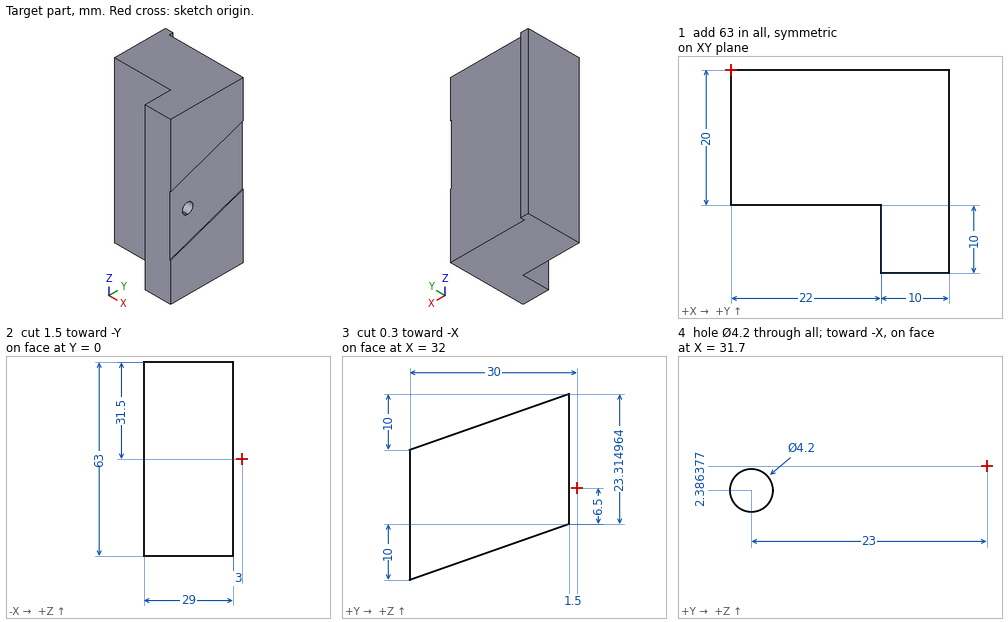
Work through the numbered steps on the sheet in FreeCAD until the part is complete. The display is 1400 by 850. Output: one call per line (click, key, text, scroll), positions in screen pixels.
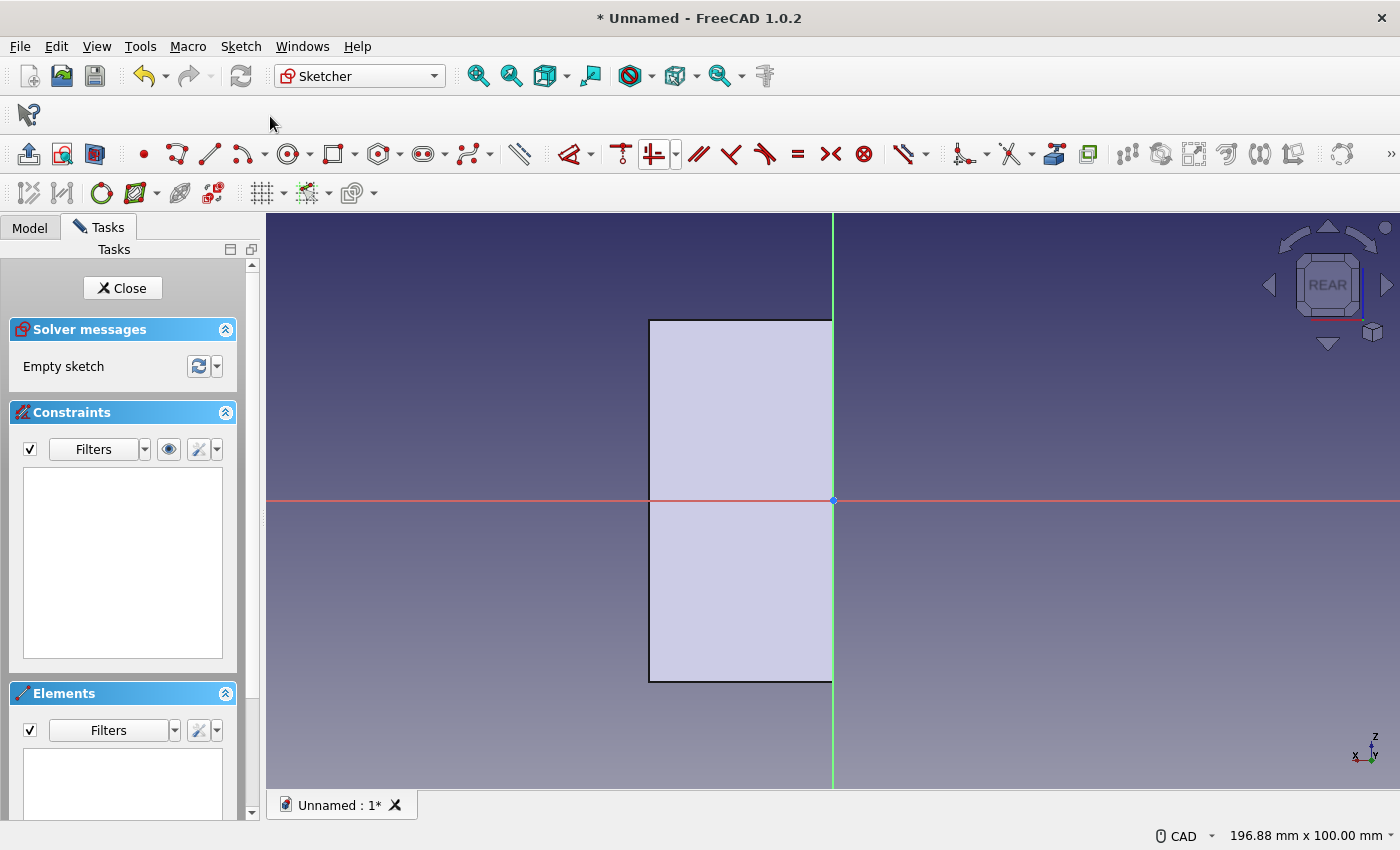
click(332, 154)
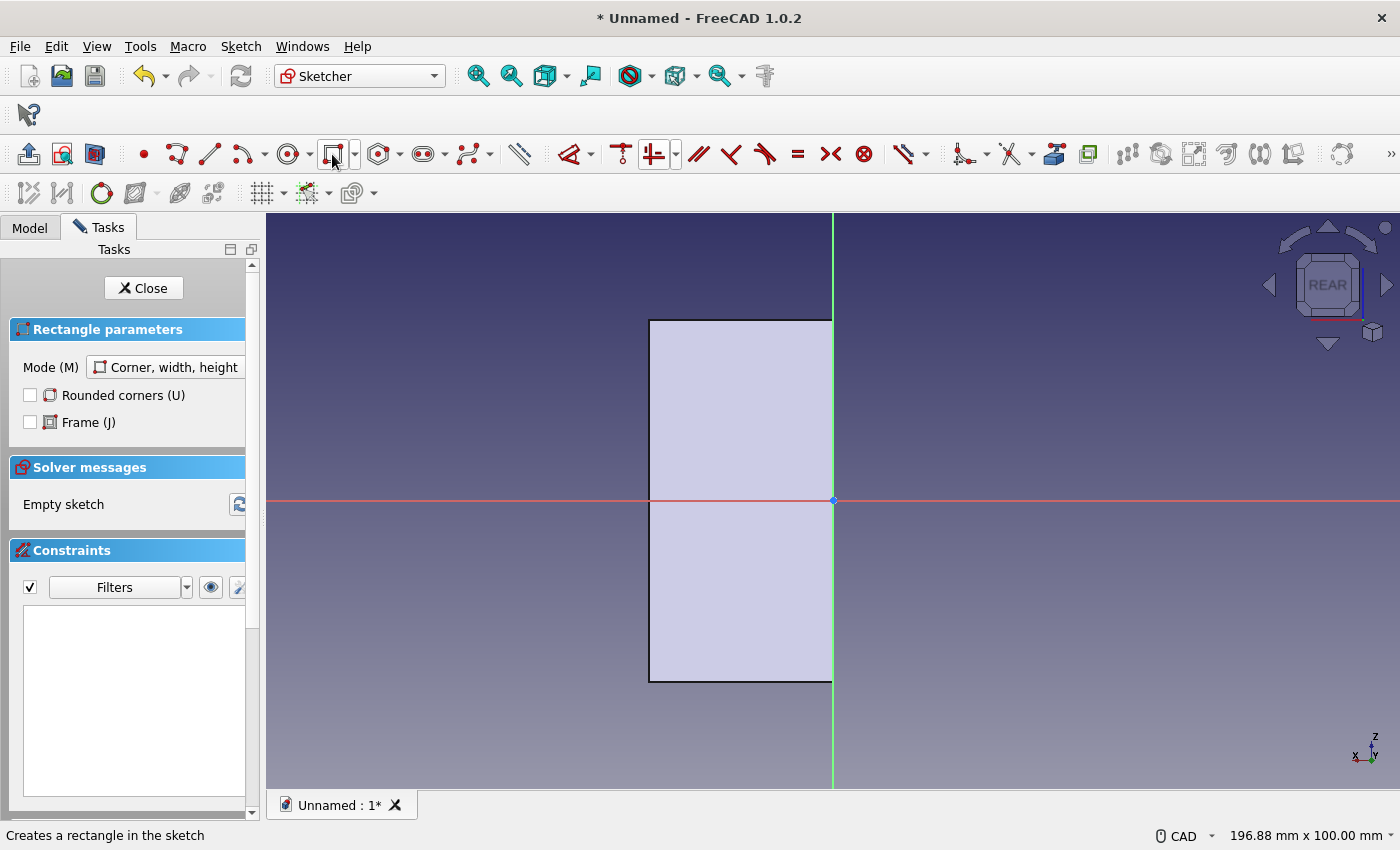
click(649, 320)
click(816, 682)
key(Escape)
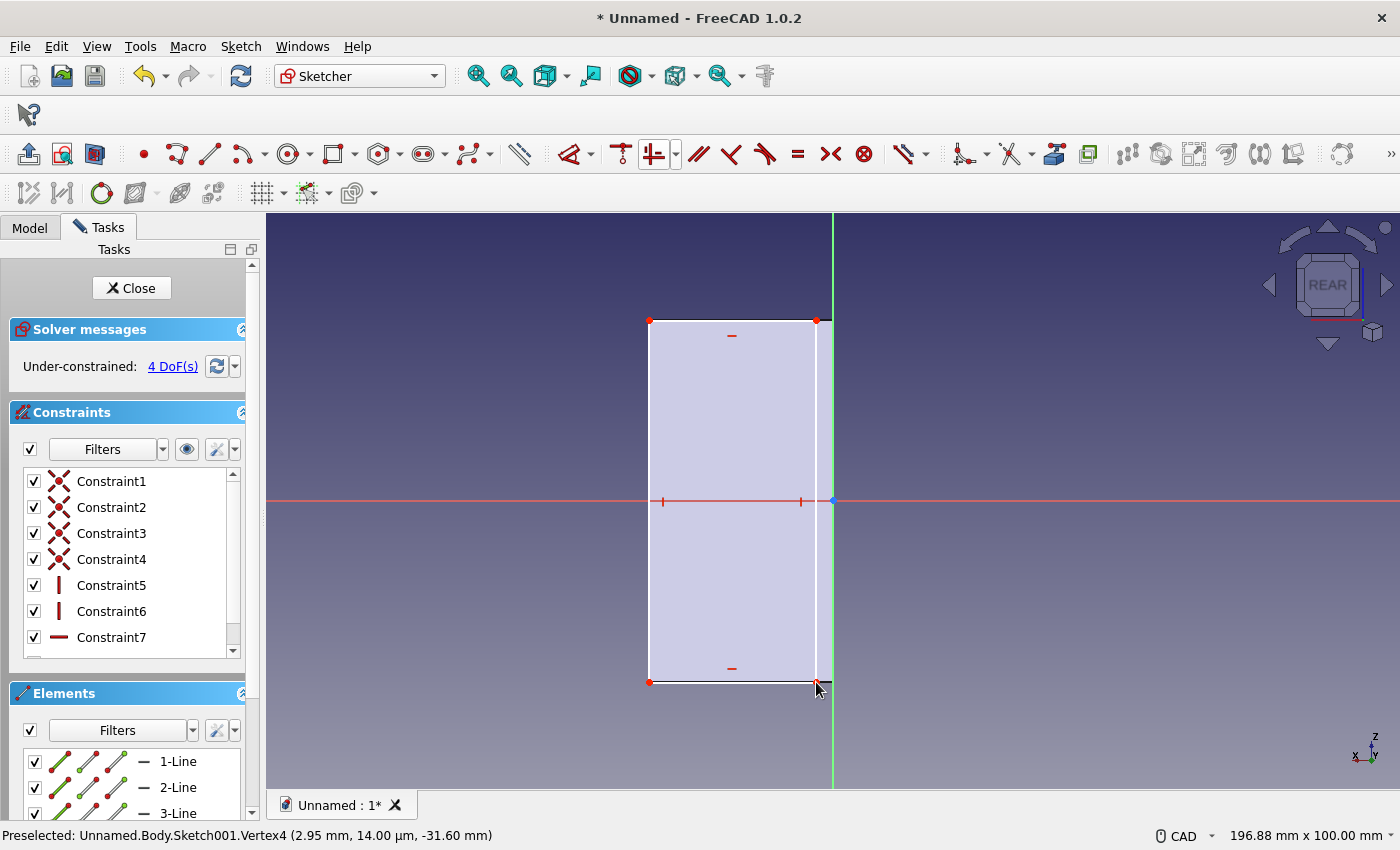
click(568, 154)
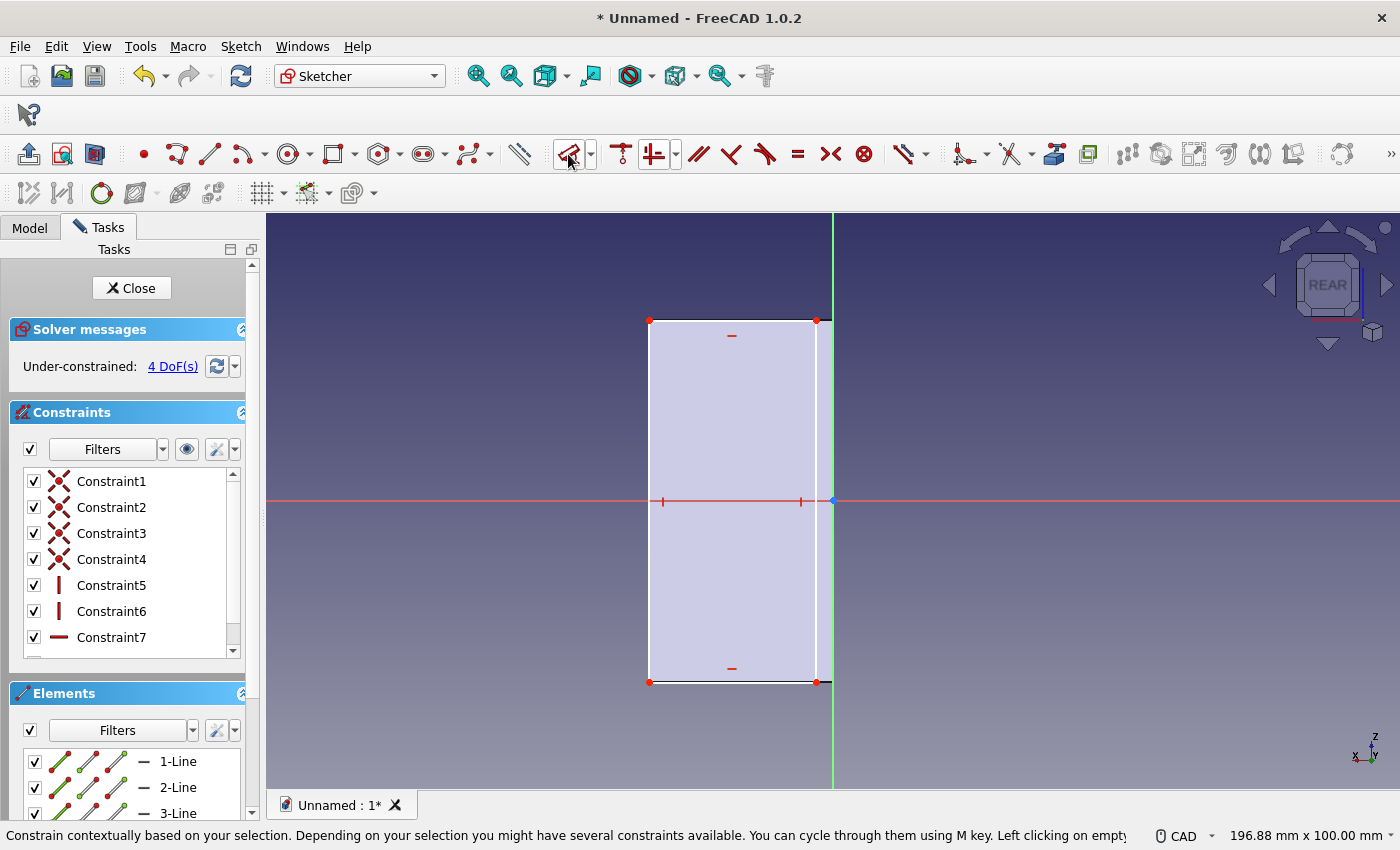
click(649, 430)
click(615, 419)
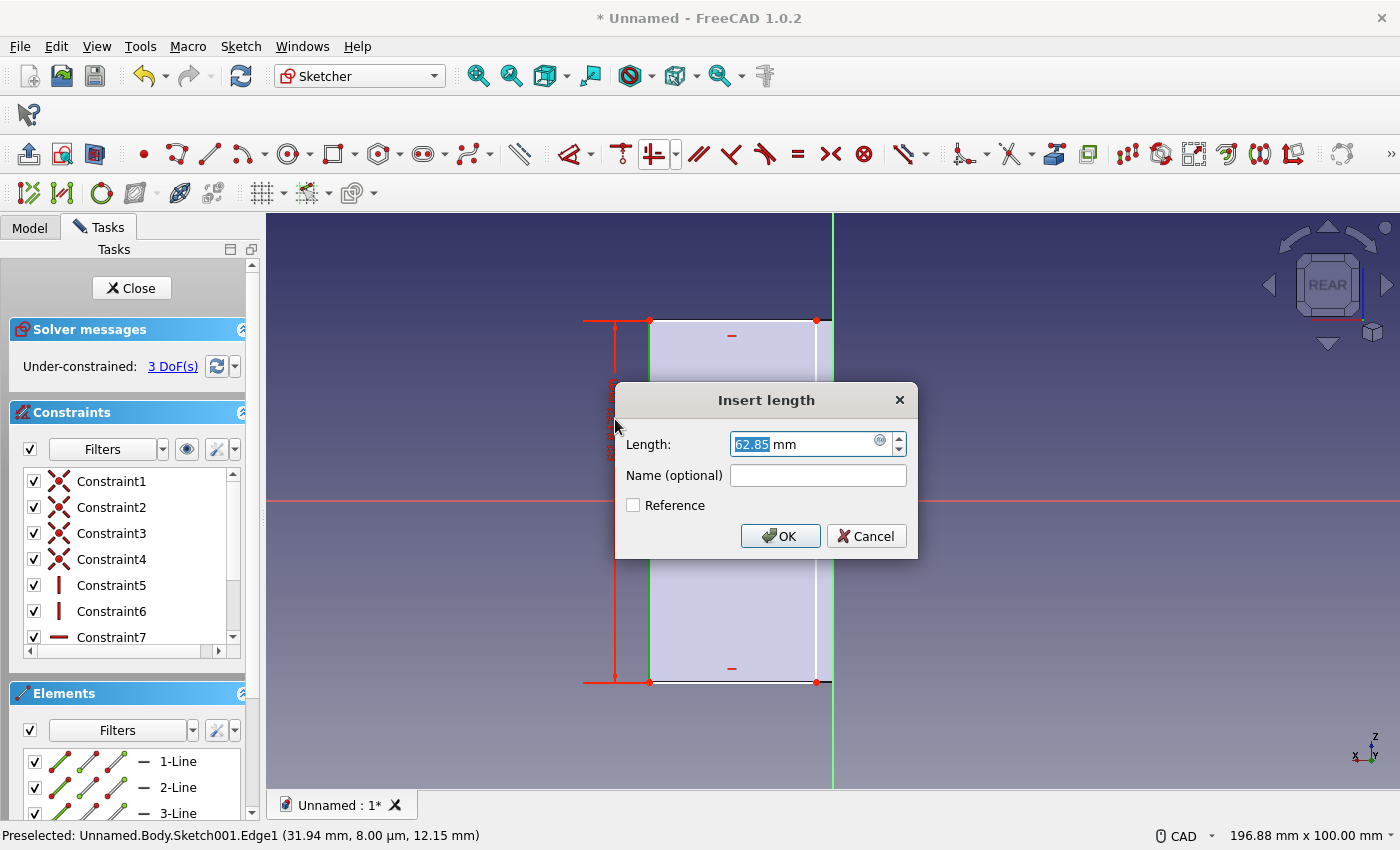
text(63)
key(Return)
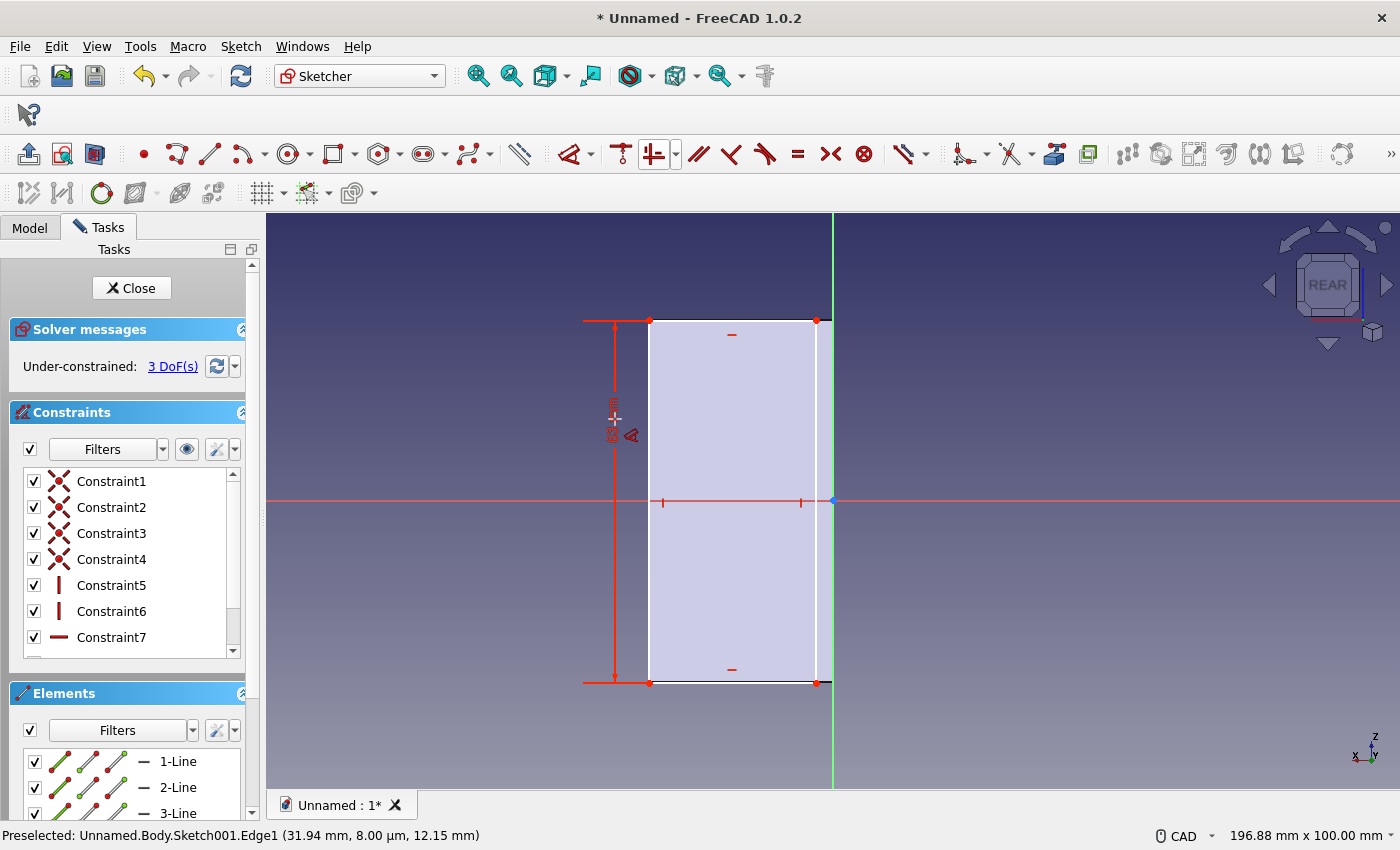
click(699, 683)
click(732, 717)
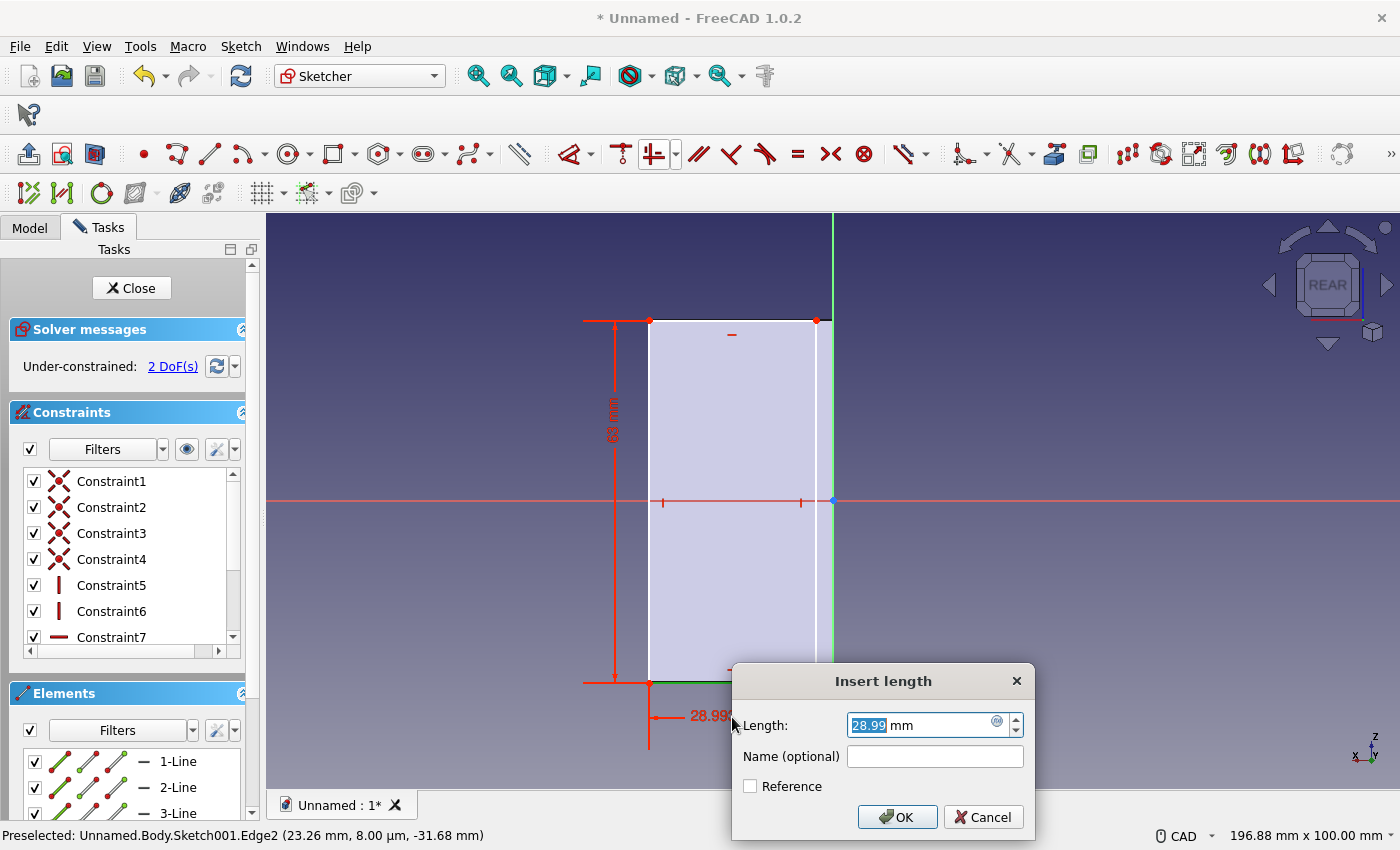
text(29)
key(Return)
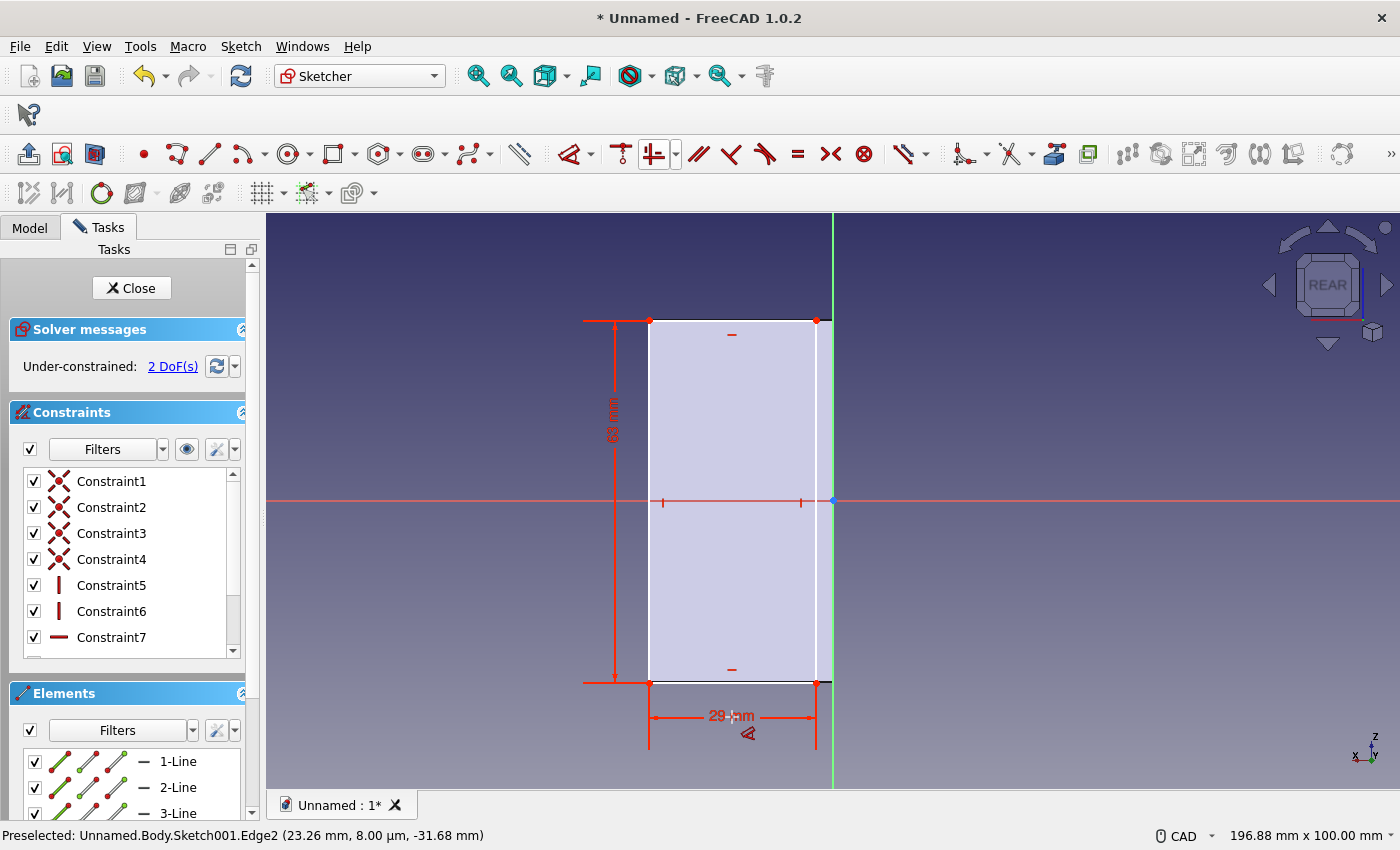
scroll(816, 683, up, 5)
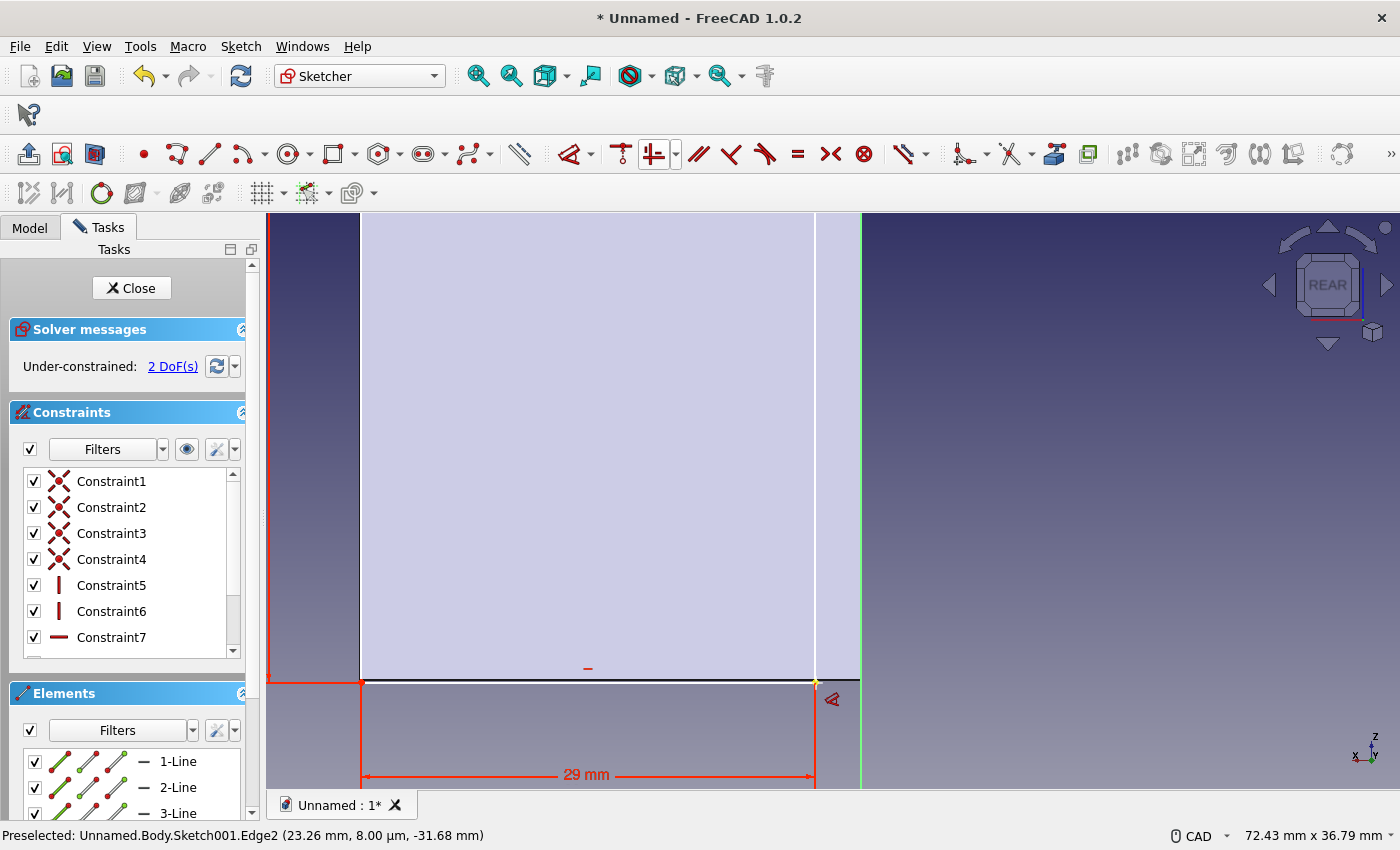
click(815, 683)
click(838, 717)